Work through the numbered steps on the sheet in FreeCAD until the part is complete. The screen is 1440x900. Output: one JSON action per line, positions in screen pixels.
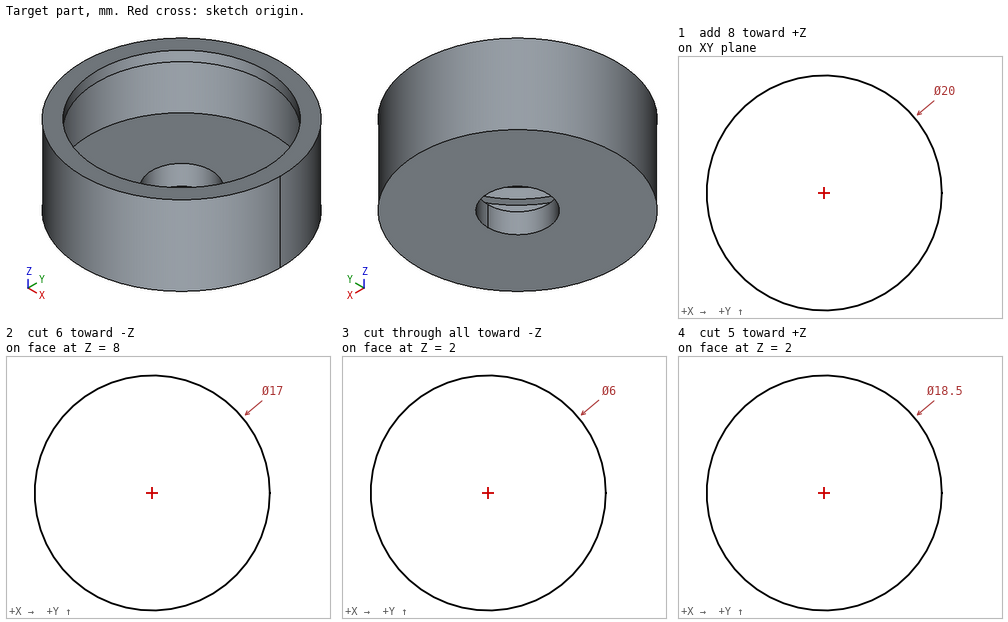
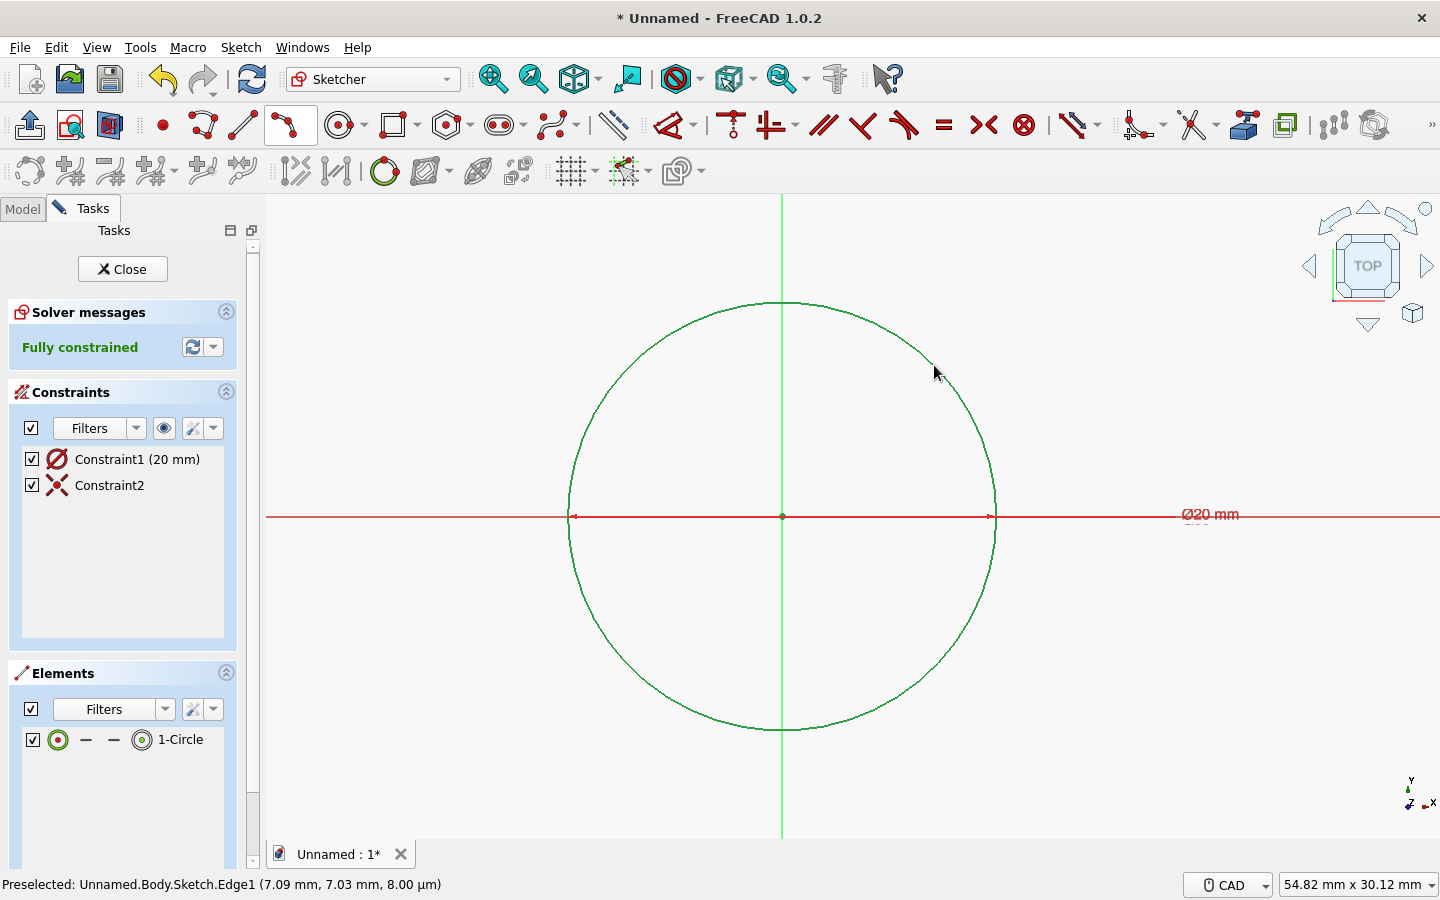
{"action": "left_click", "coordinate": [123, 269]}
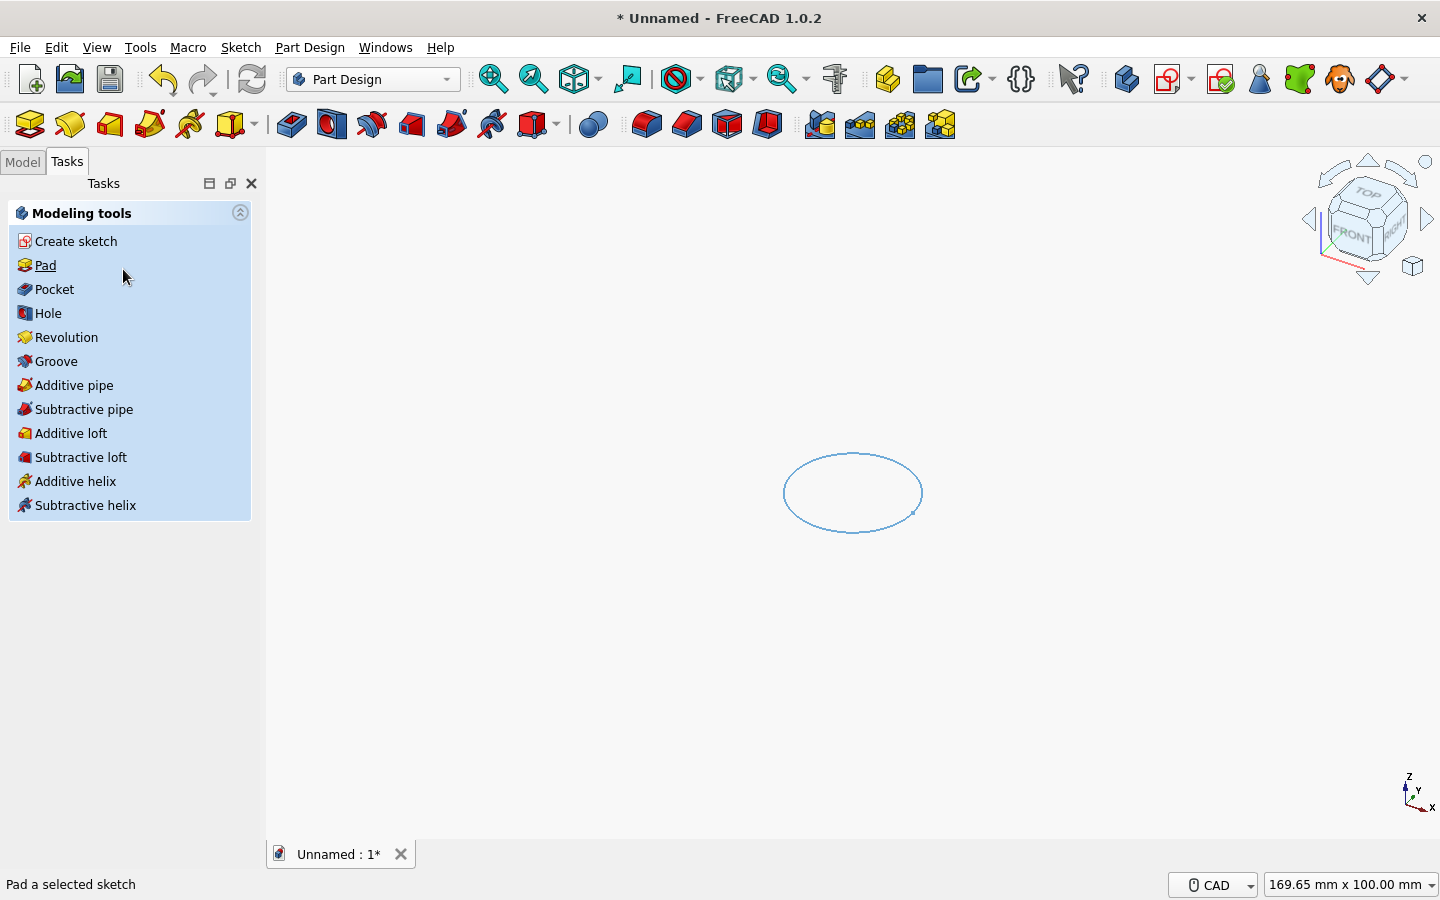
{"action": "left_click", "coordinate": [30, 124]}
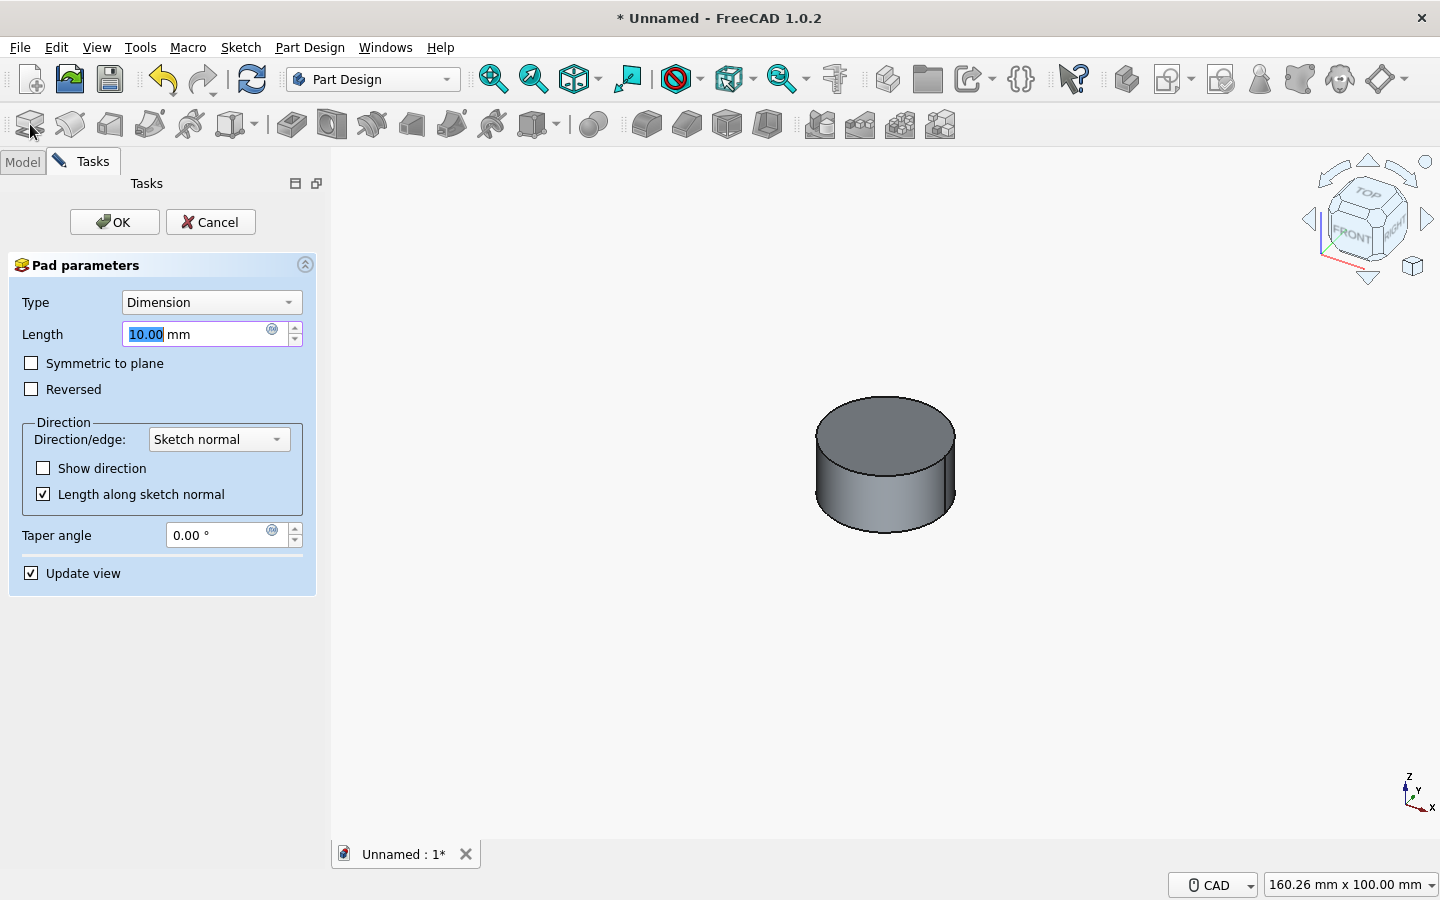
{"action": "type", "text": "8"}
{"action": "key", "text": "Tab"}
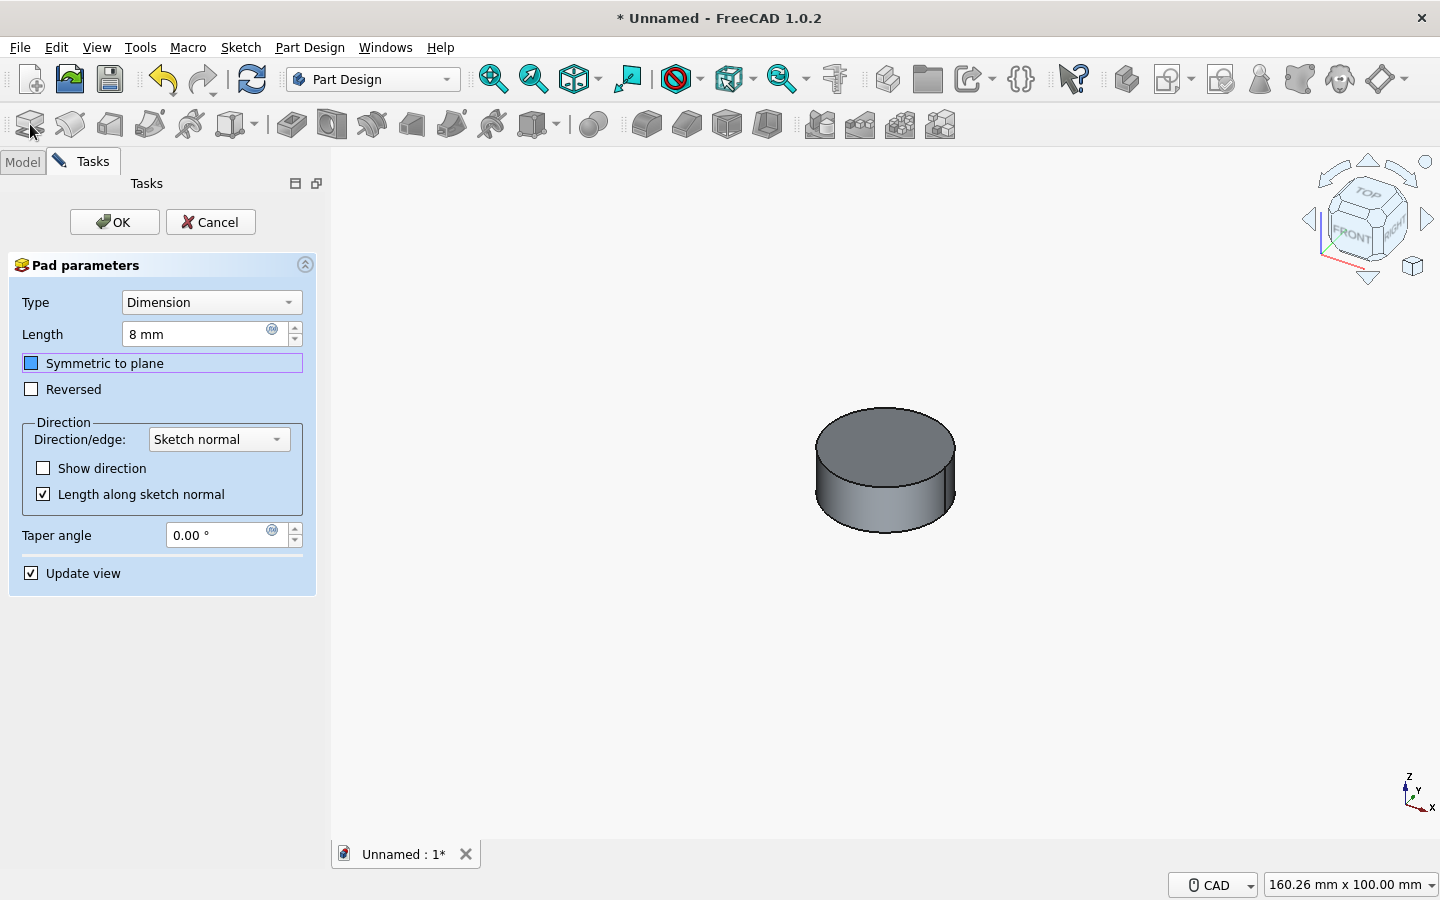
{"action": "left_click", "coordinate": [115, 222]}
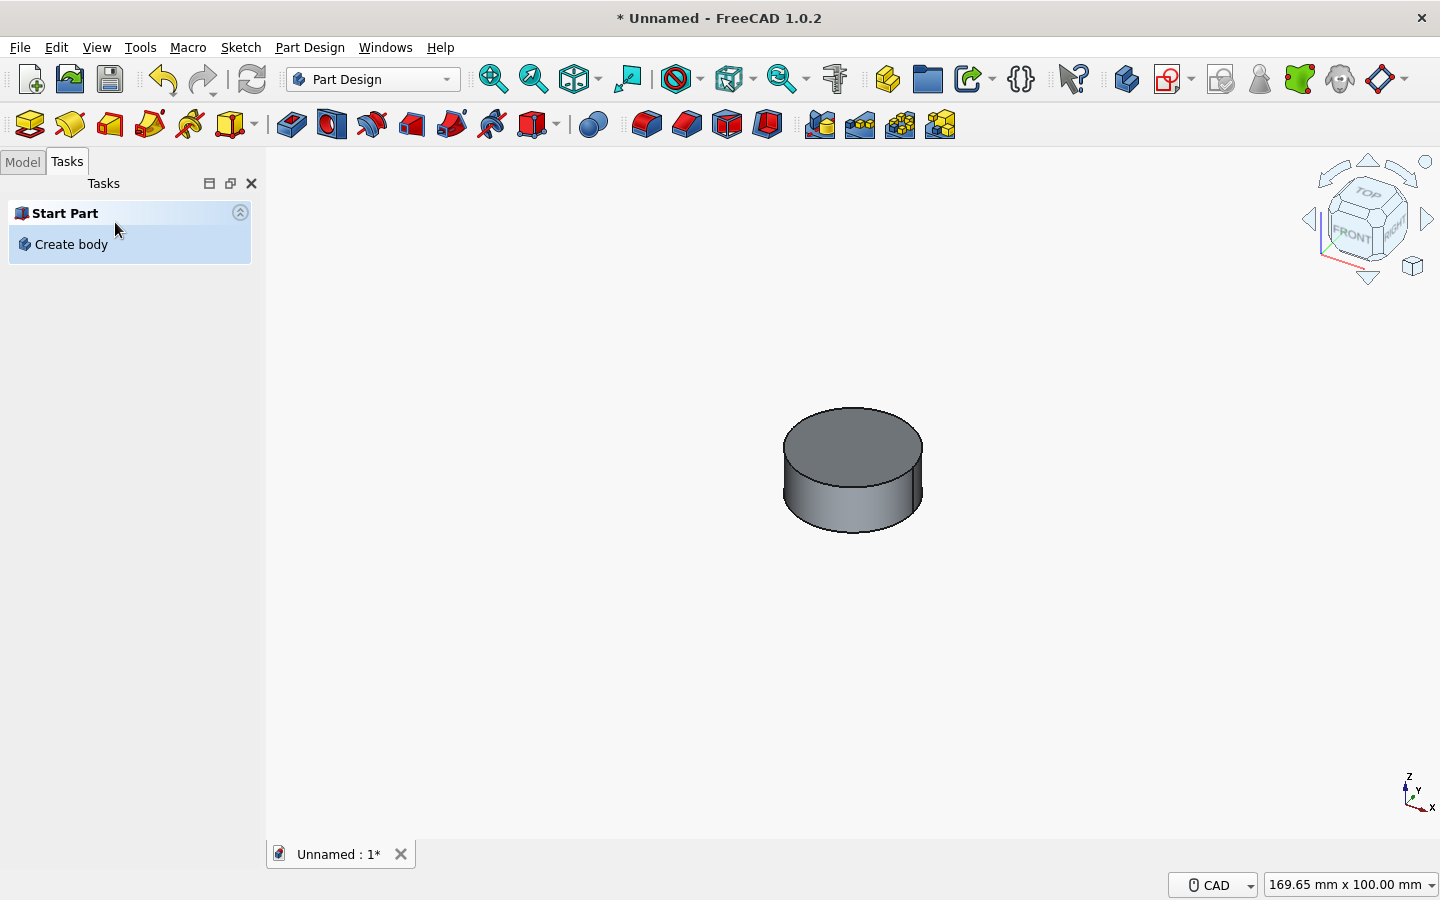
{"action": "left_click", "coordinate": [494, 80]}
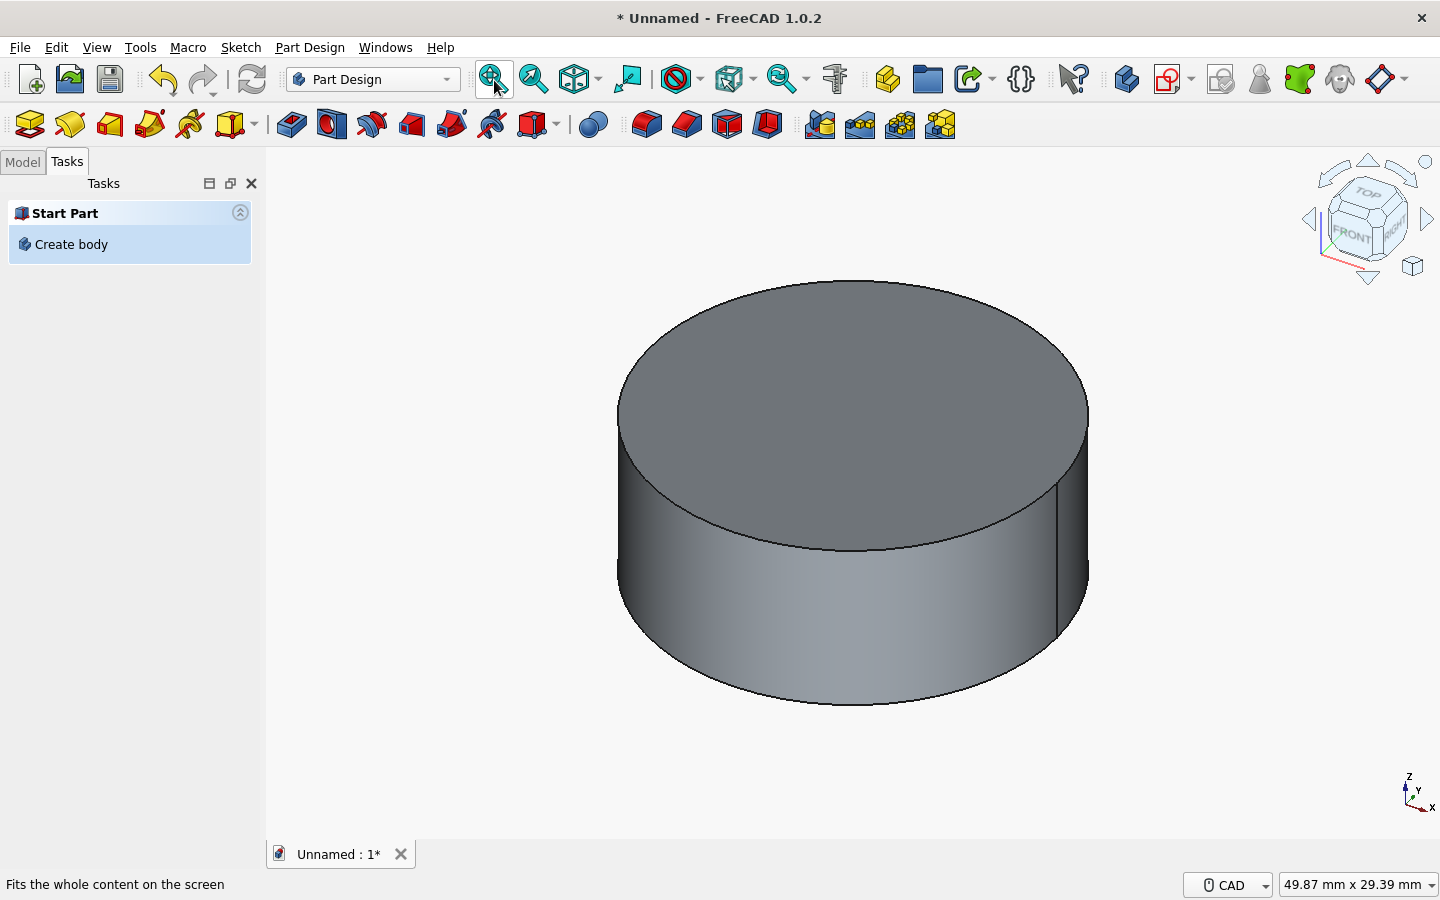
{"action": "left_click", "coordinate": [853, 415]}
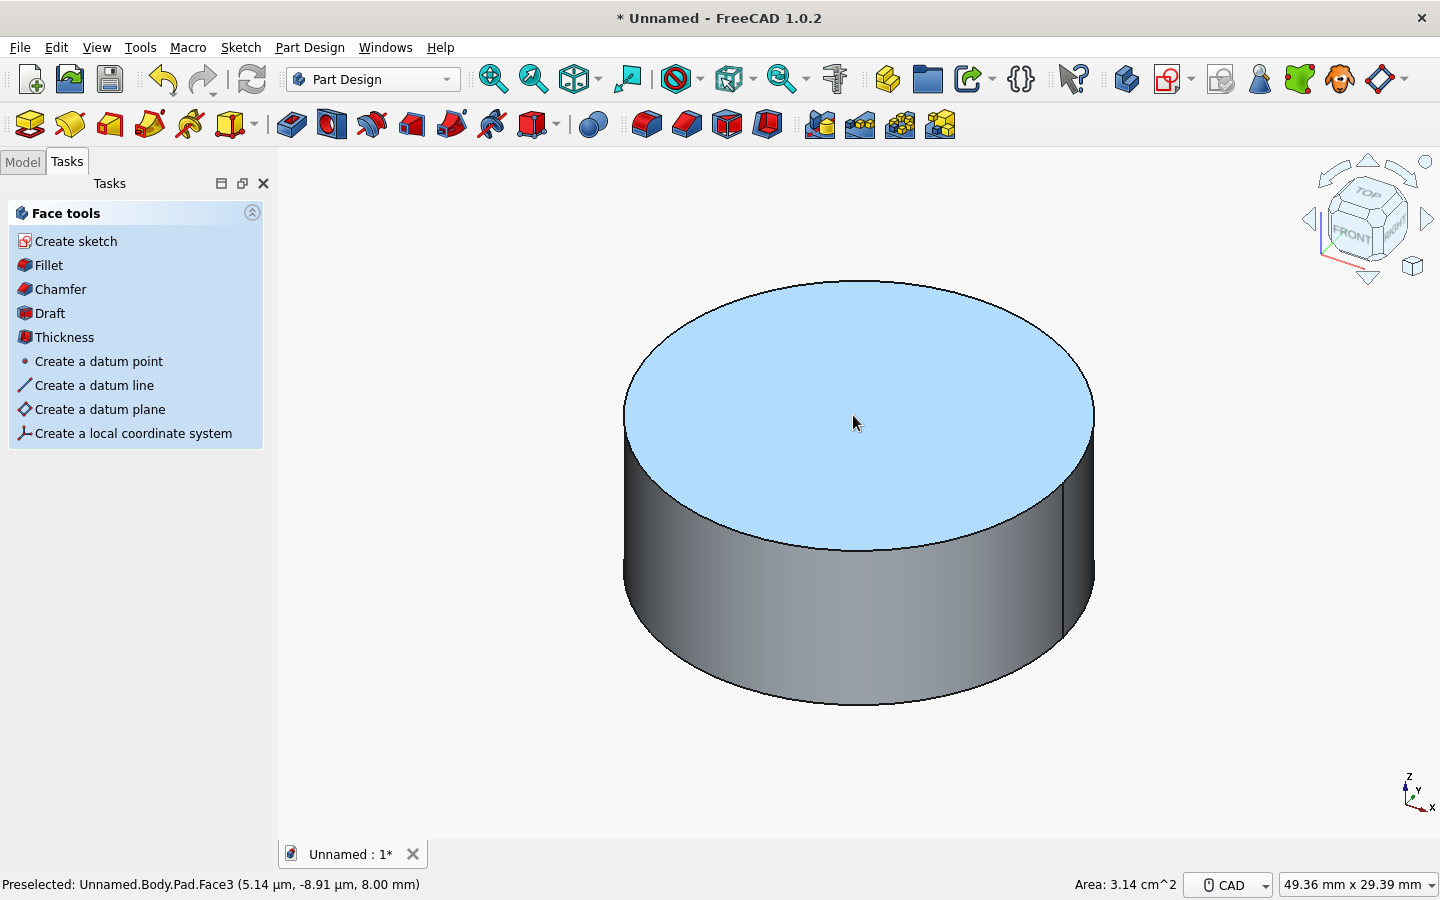
{"action": "left_click", "coordinate": [1168, 80]}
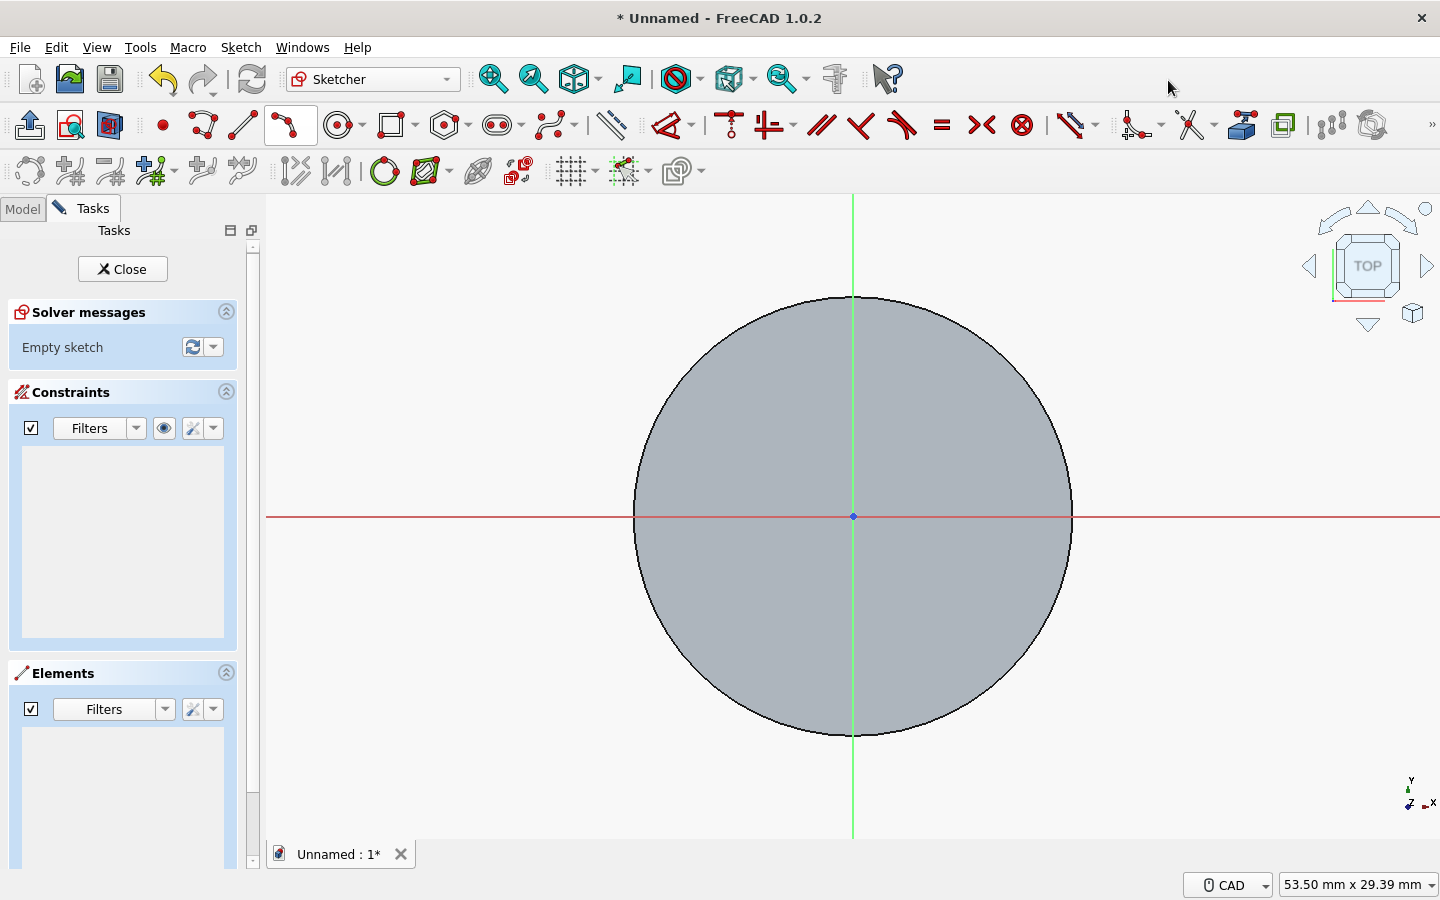
{"action": "left_click", "coordinate": [338, 126]}